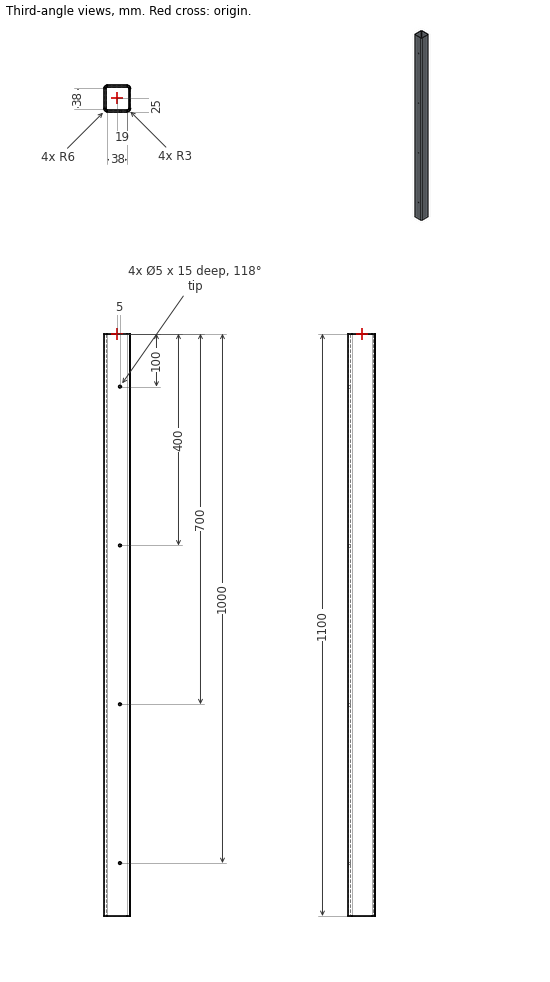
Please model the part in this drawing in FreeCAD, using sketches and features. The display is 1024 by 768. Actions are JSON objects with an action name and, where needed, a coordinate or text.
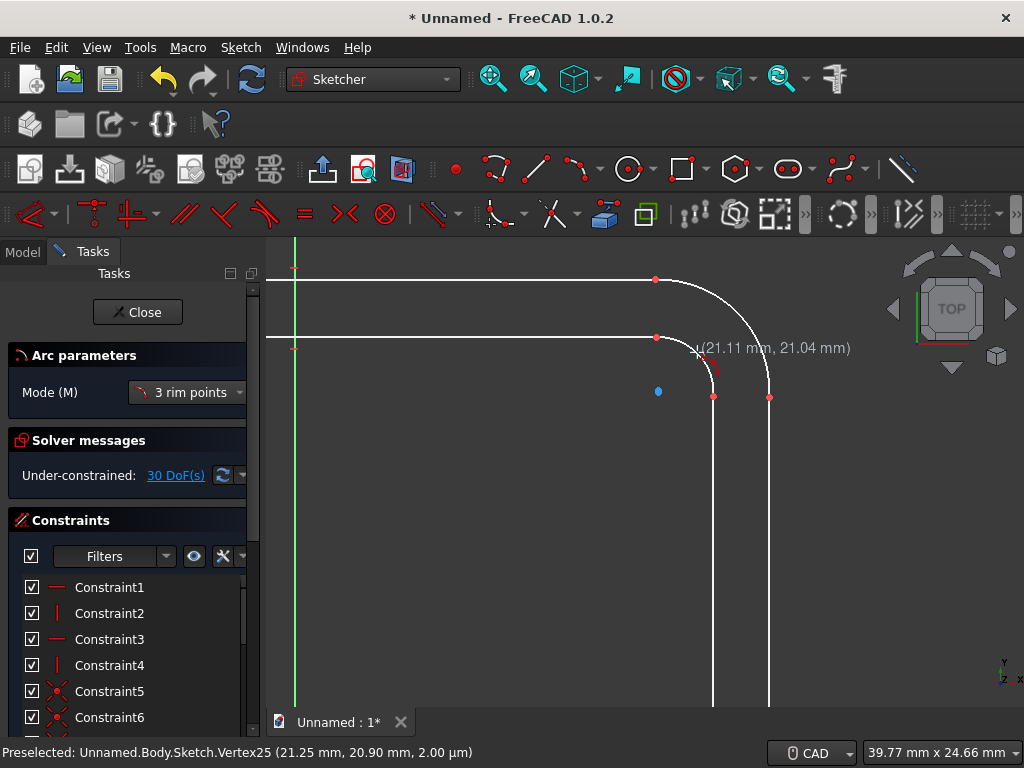
{"action": "scroll", "coordinate": [698, 350], "scroll_direction": "down", "scroll_amount": 6}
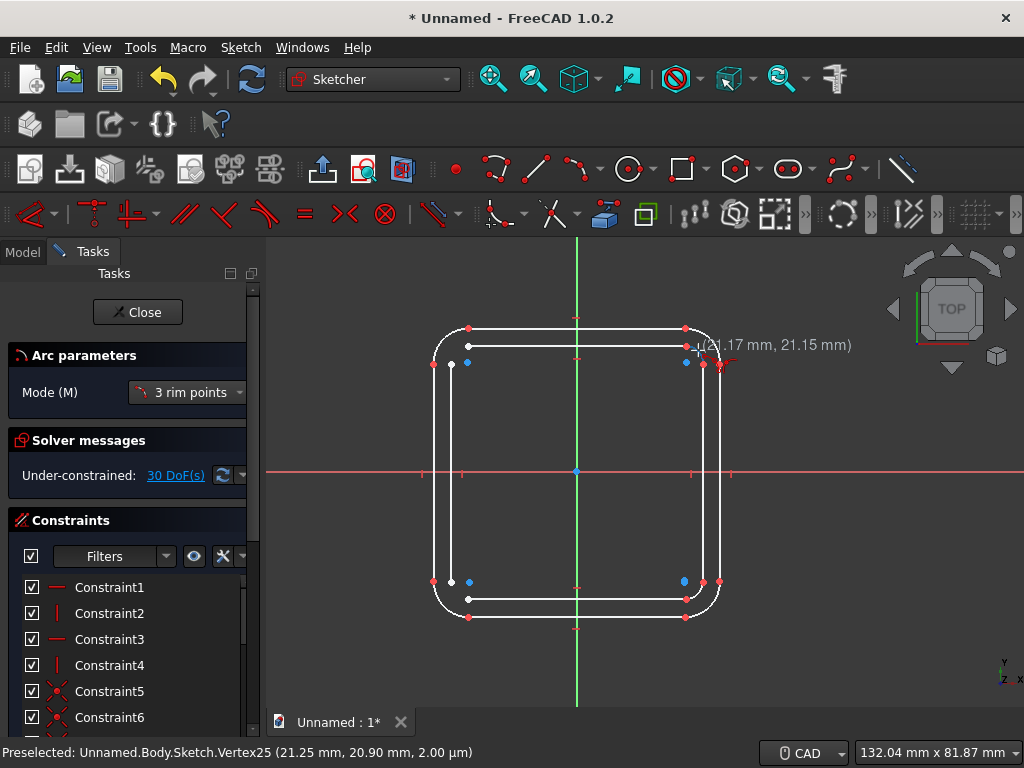
{"action": "left_click", "coordinate": [468, 346]}
{"action": "left_click", "coordinate": [451, 364]}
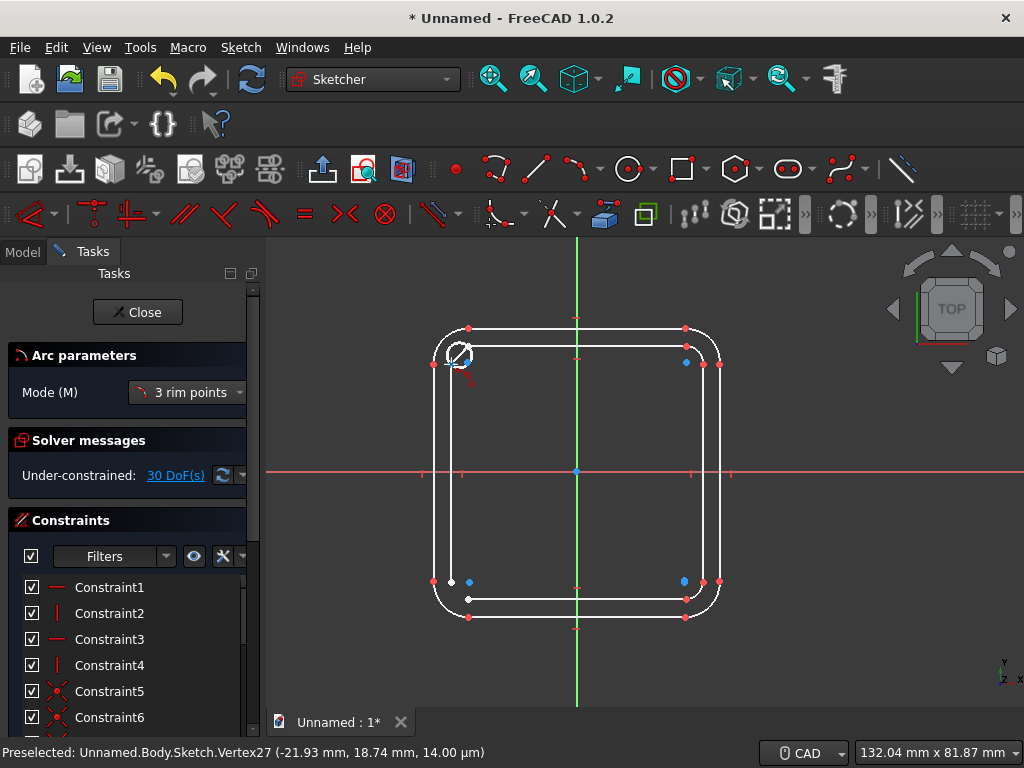
{"action": "scroll", "coordinate": [456, 351], "scroll_direction": "up", "scroll_amount": 6}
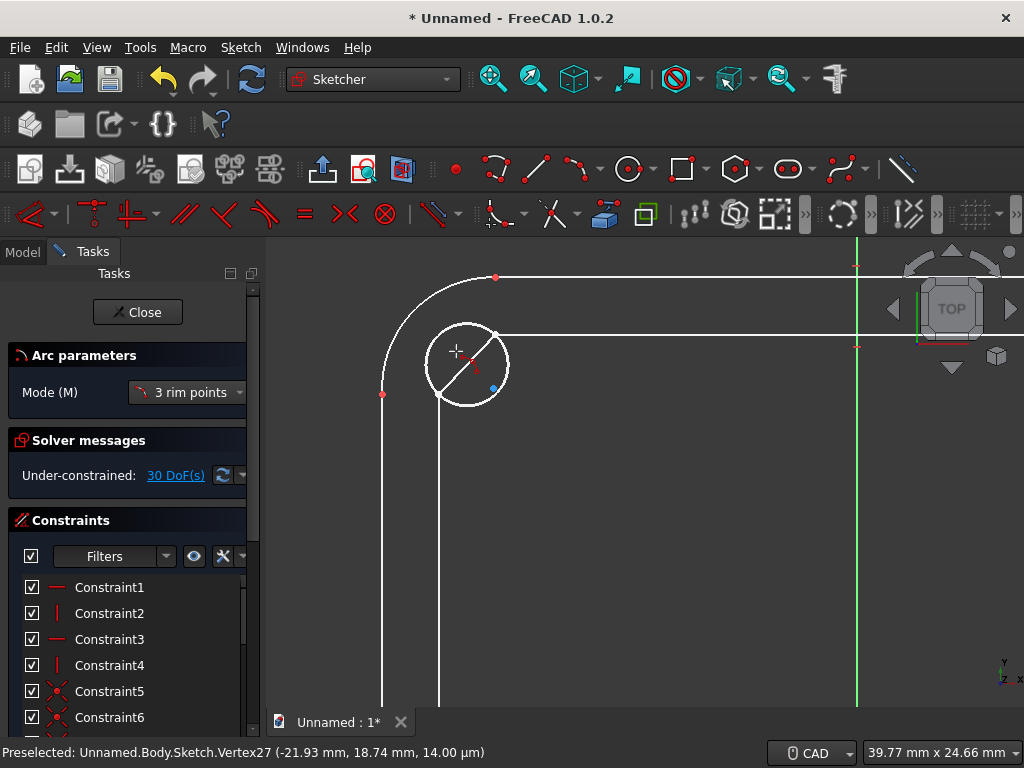
{"action": "left_click", "coordinate": [454, 349]}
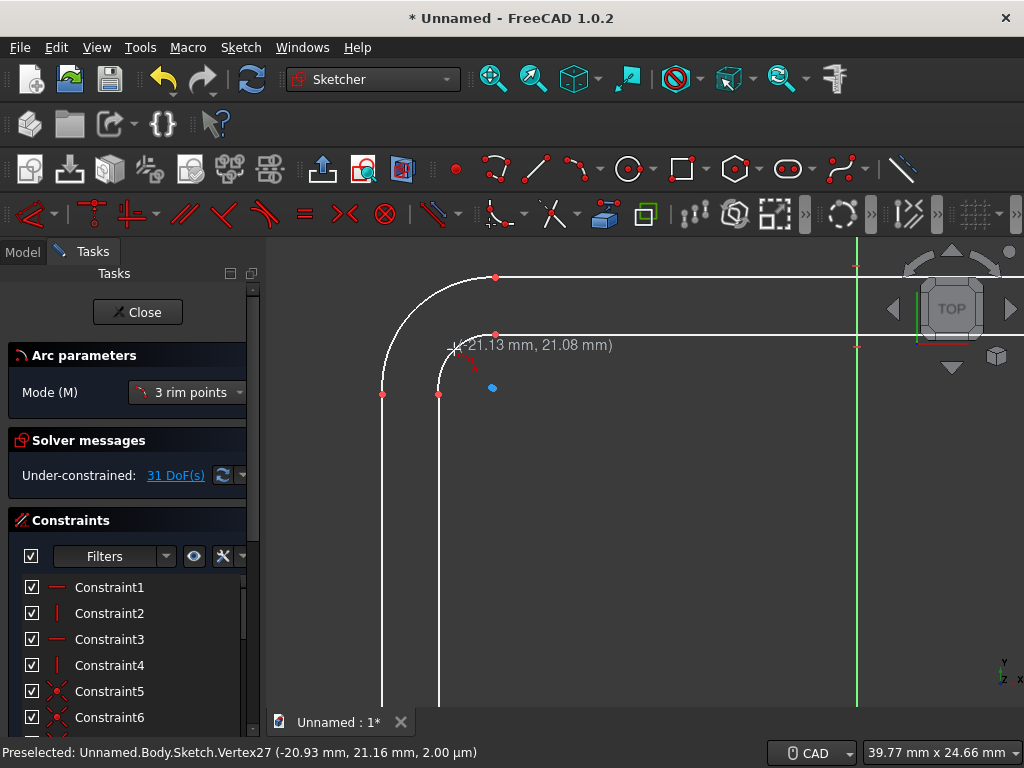
{"action": "scroll", "coordinate": [456, 351], "scroll_direction": "down", "scroll_amount": 6}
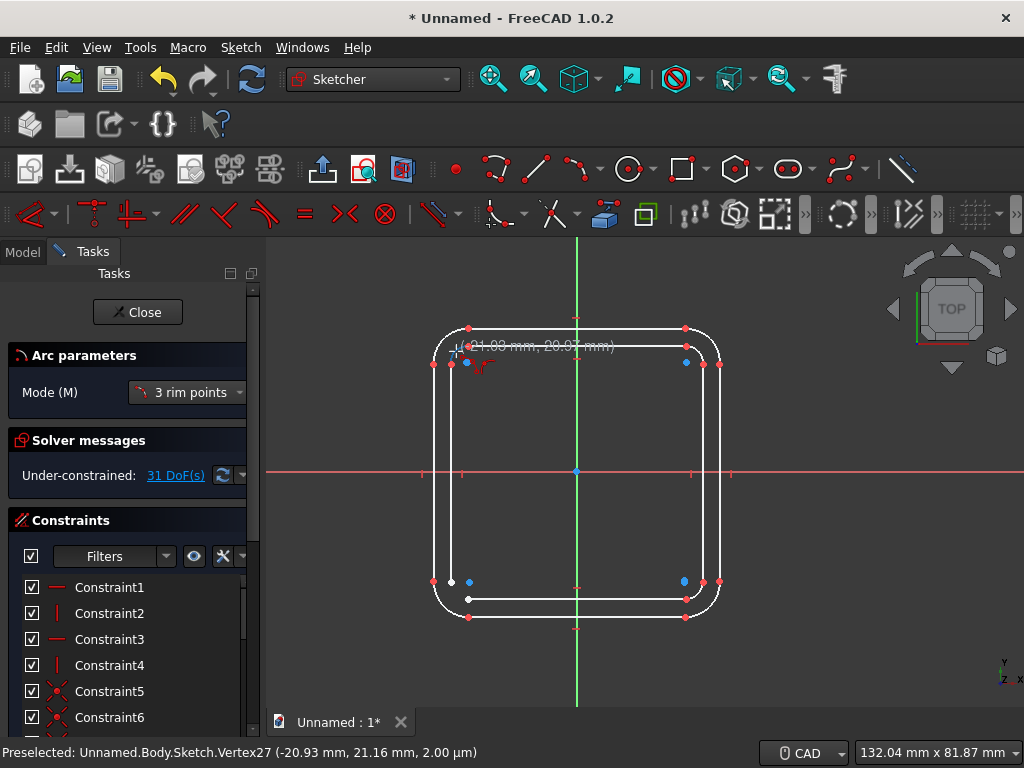
{"action": "left_click", "coordinate": [451, 582]}
{"action": "left_click", "coordinate": [468, 599]}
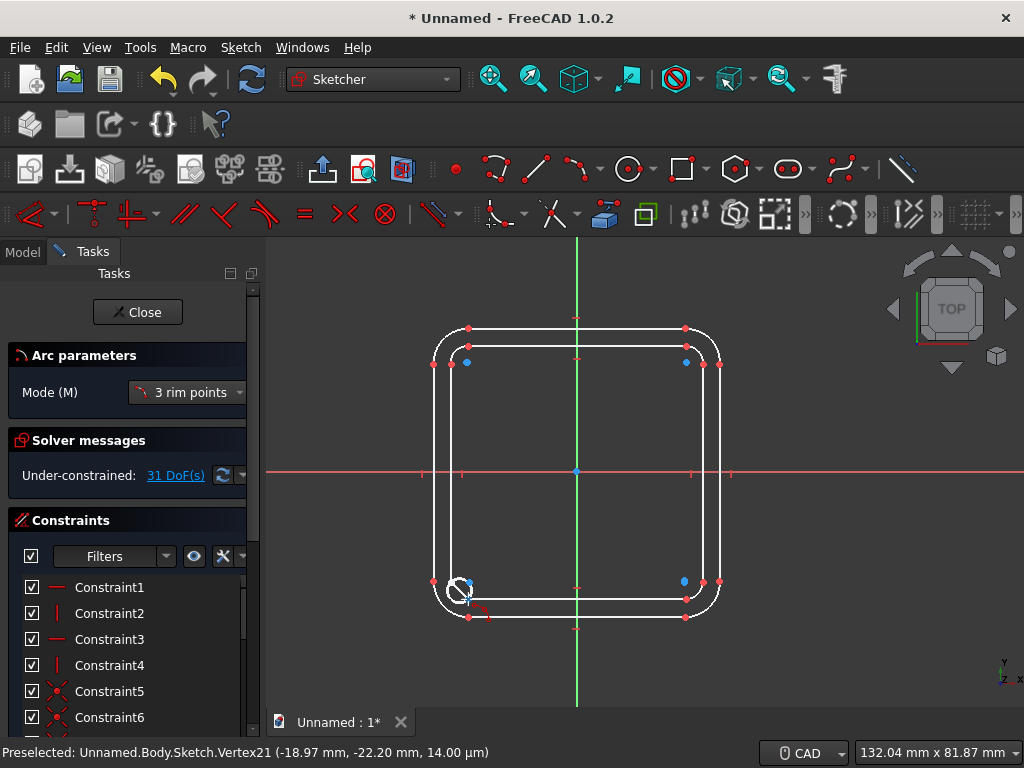
{"action": "scroll", "coordinate": [456, 593], "scroll_direction": "up", "scroll_amount": 6}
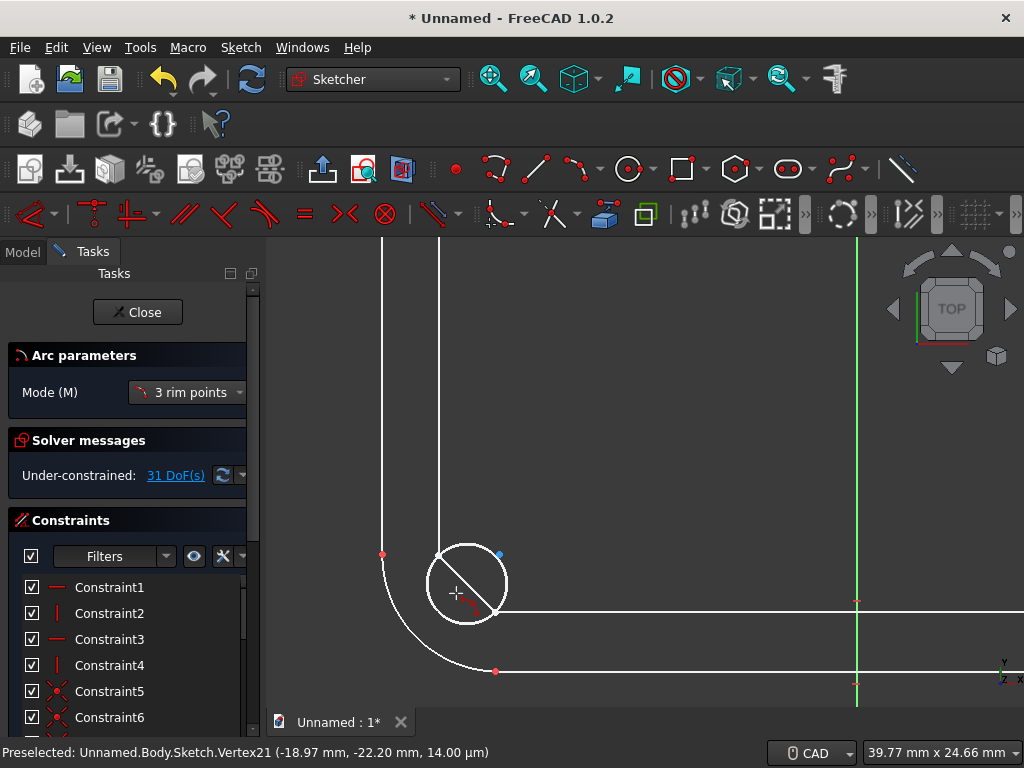
{"action": "left_click", "coordinate": [454, 592]}
{"action": "key", "text": "Escape"}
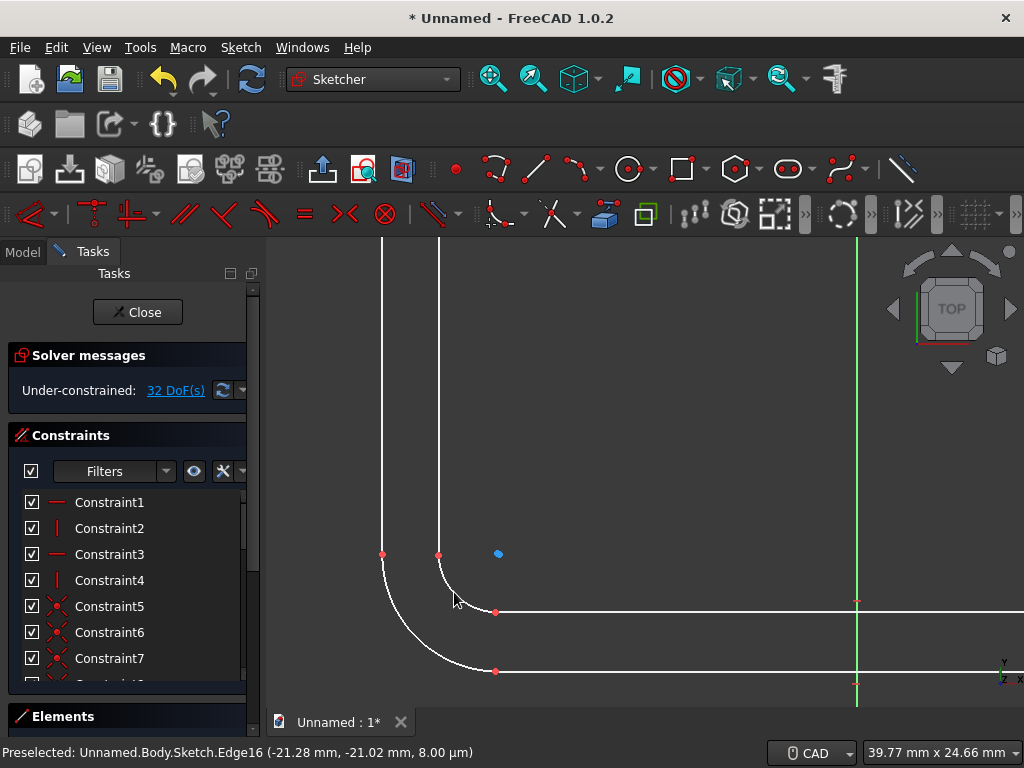
{"action": "scroll", "coordinate": [456, 594], "scroll_direction": "down", "scroll_amount": 6}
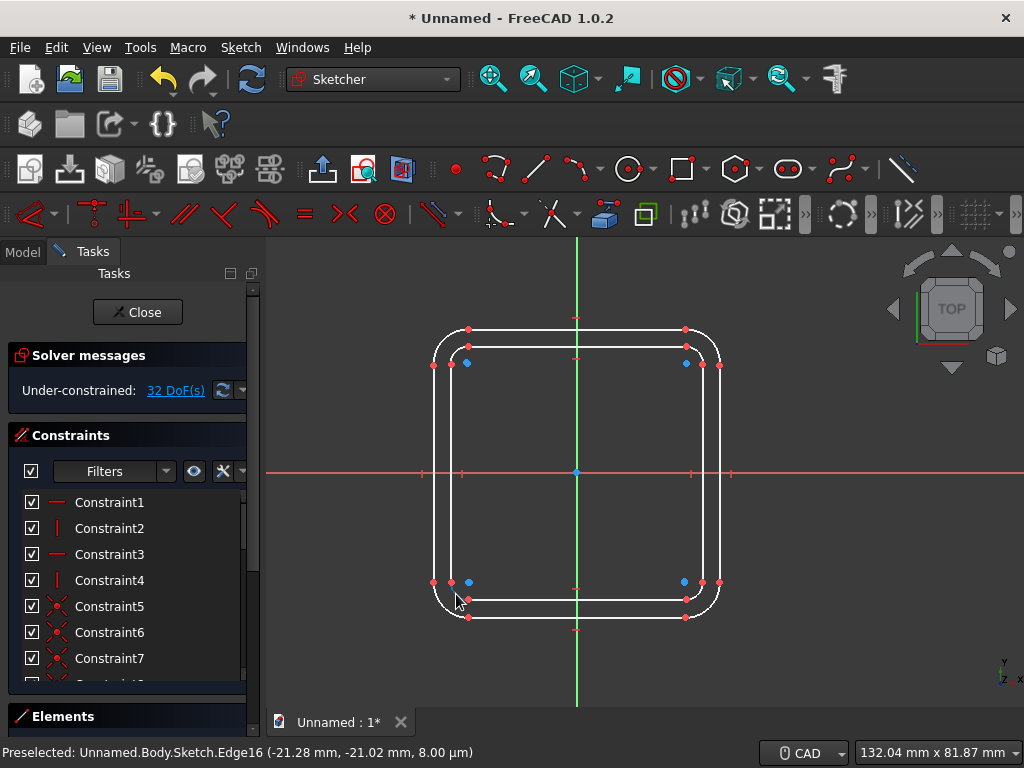
{"action": "left_click", "coordinate": [533, 618]}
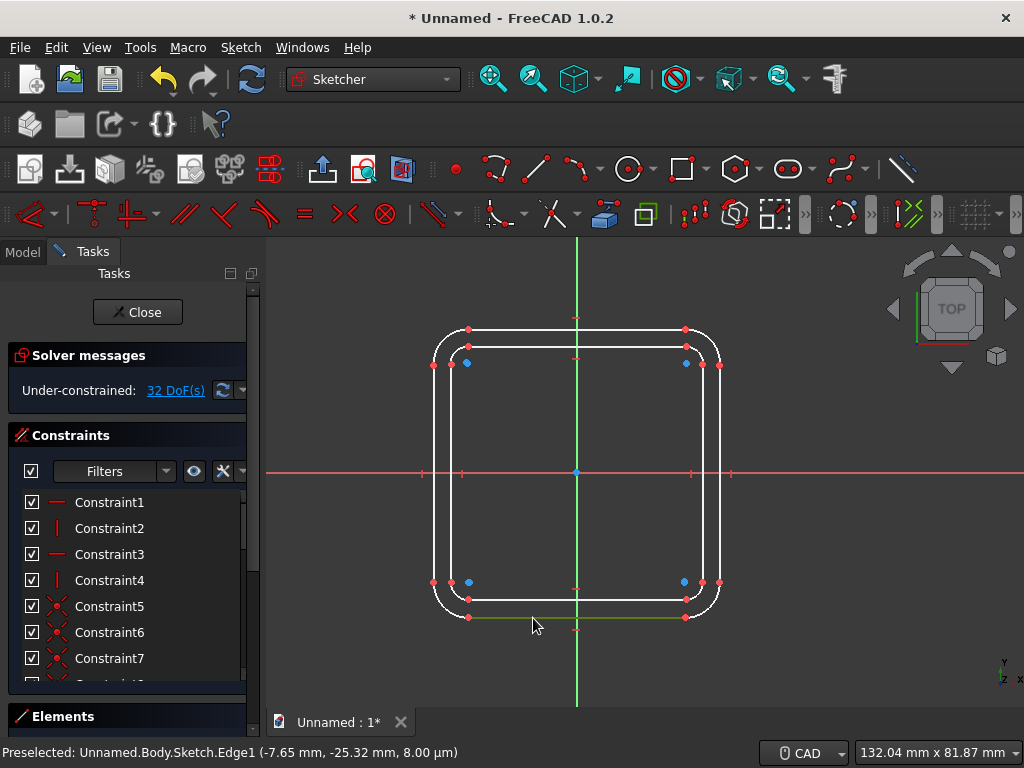
{"action": "left_click", "coordinate": [438, 598]}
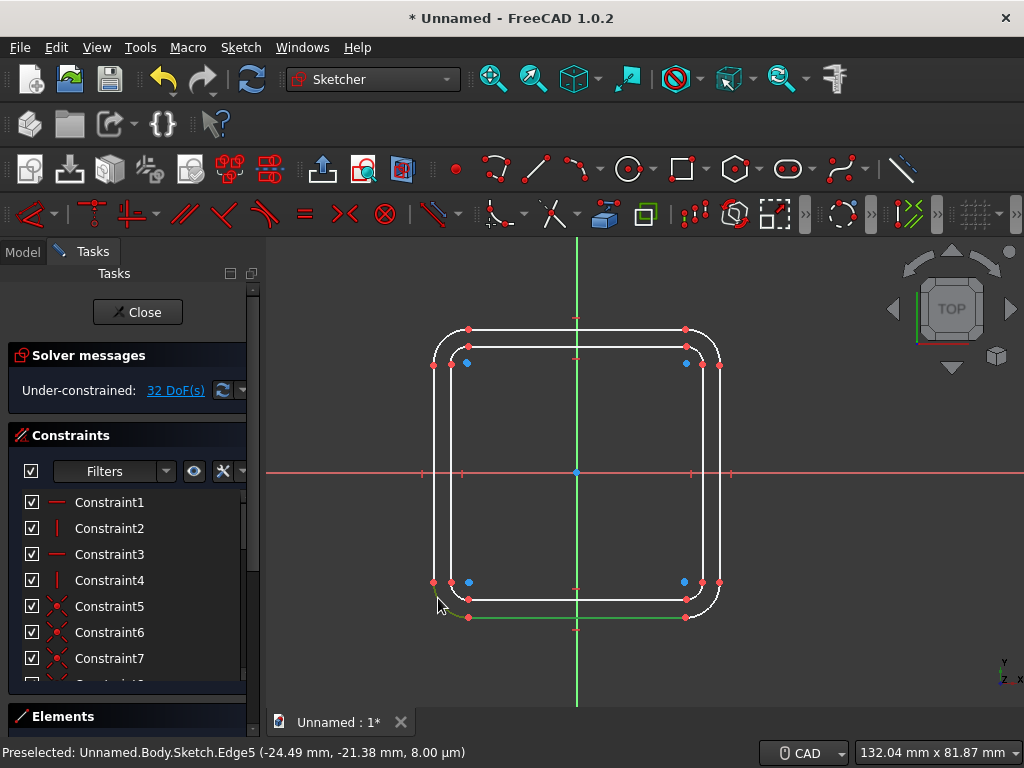
{"action": "key", "text": "t"}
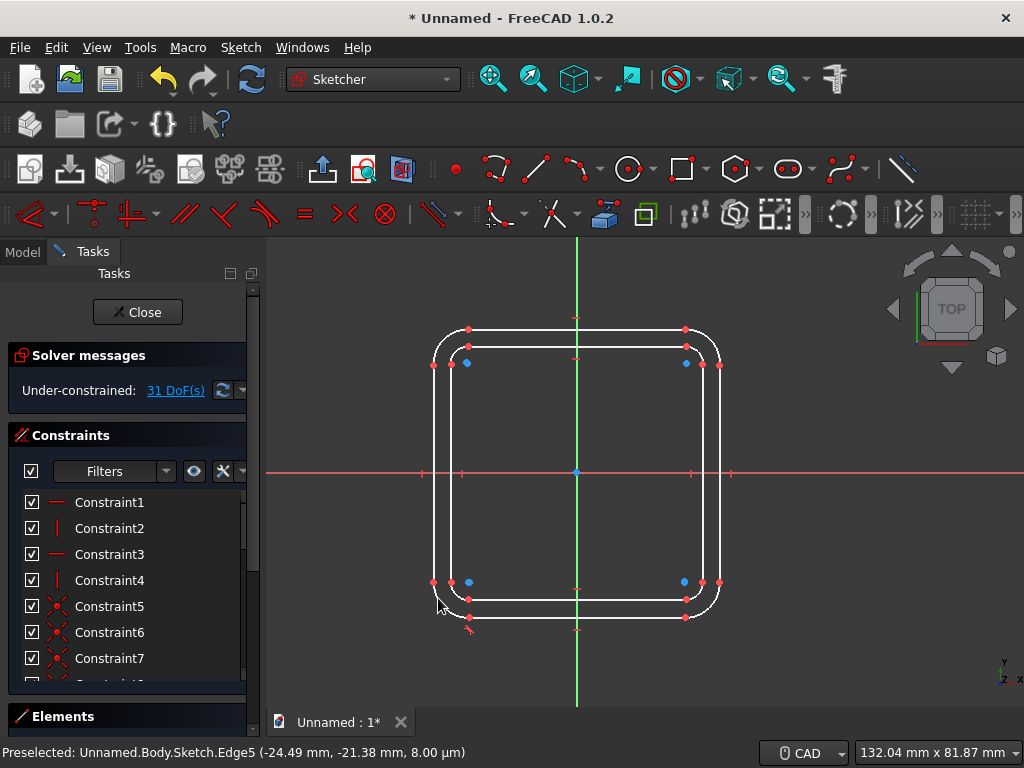
{"action": "left_click", "coordinate": [621, 618]}